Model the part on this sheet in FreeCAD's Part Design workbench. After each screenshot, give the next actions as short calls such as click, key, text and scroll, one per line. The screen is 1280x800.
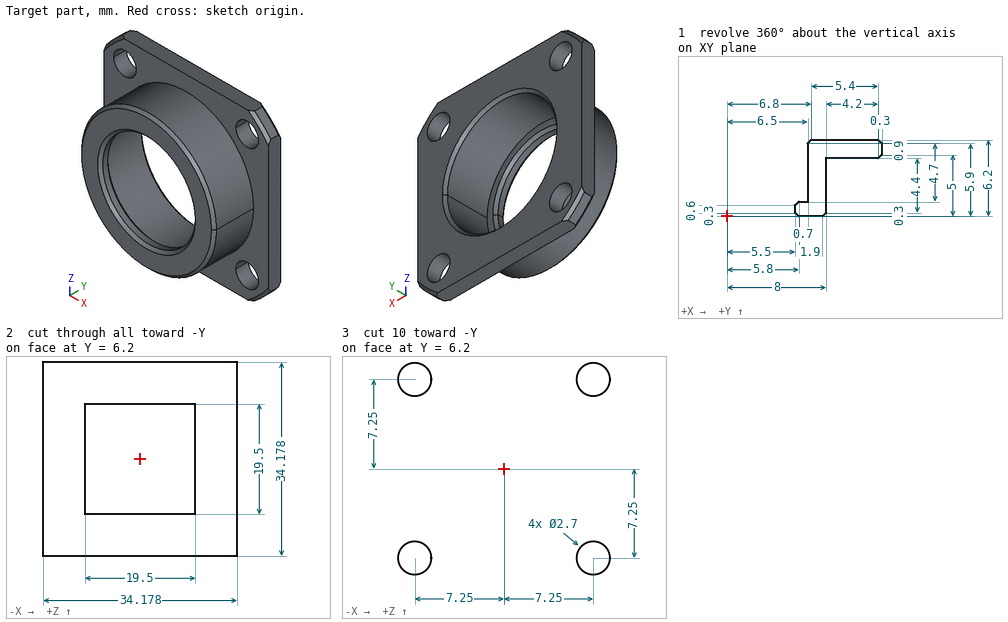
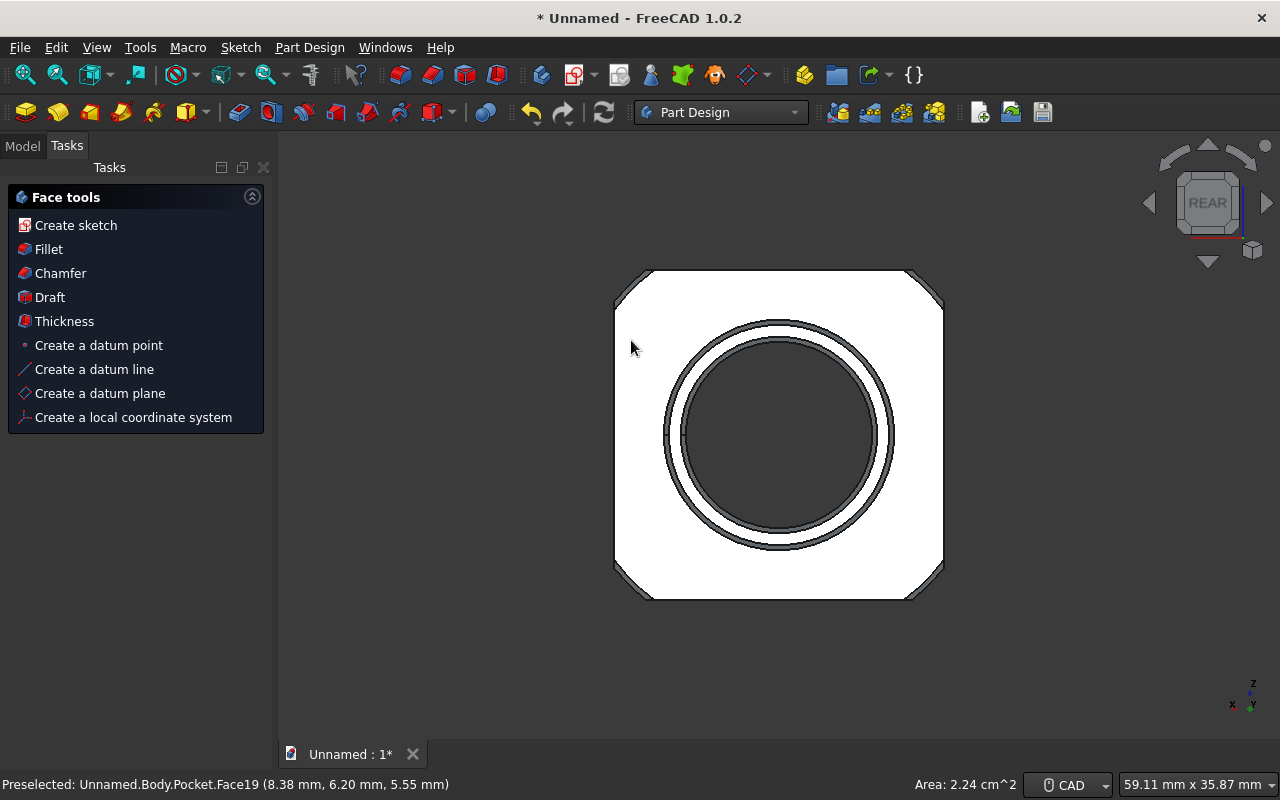
click(574, 76)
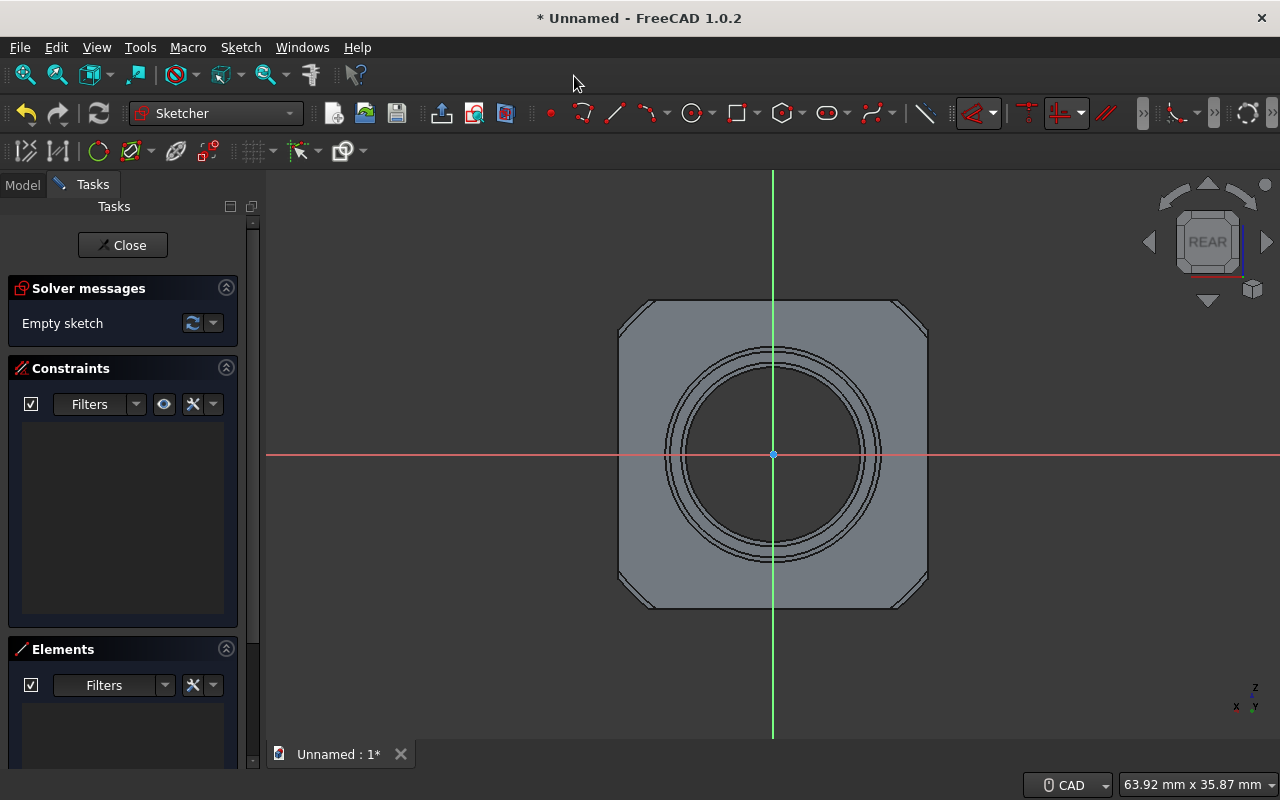
click(692, 114)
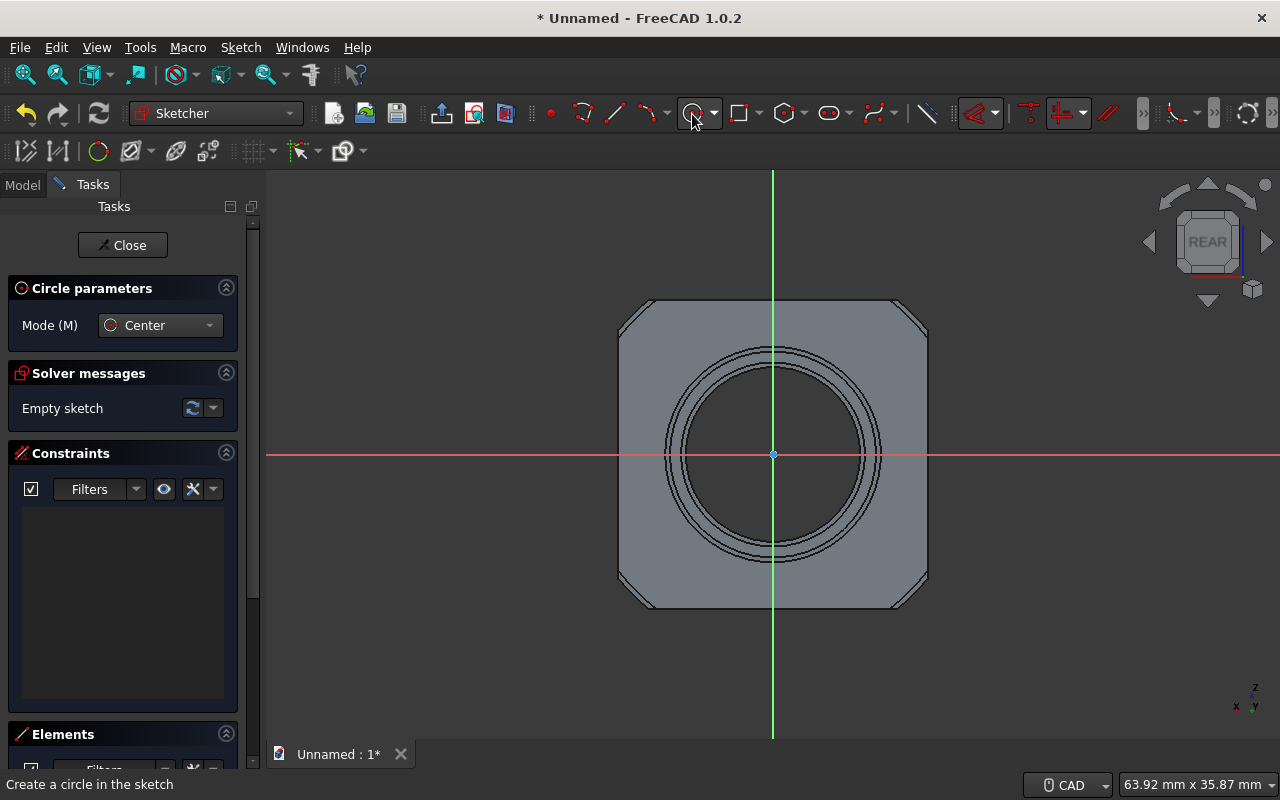
click(888, 570)
click(903, 554)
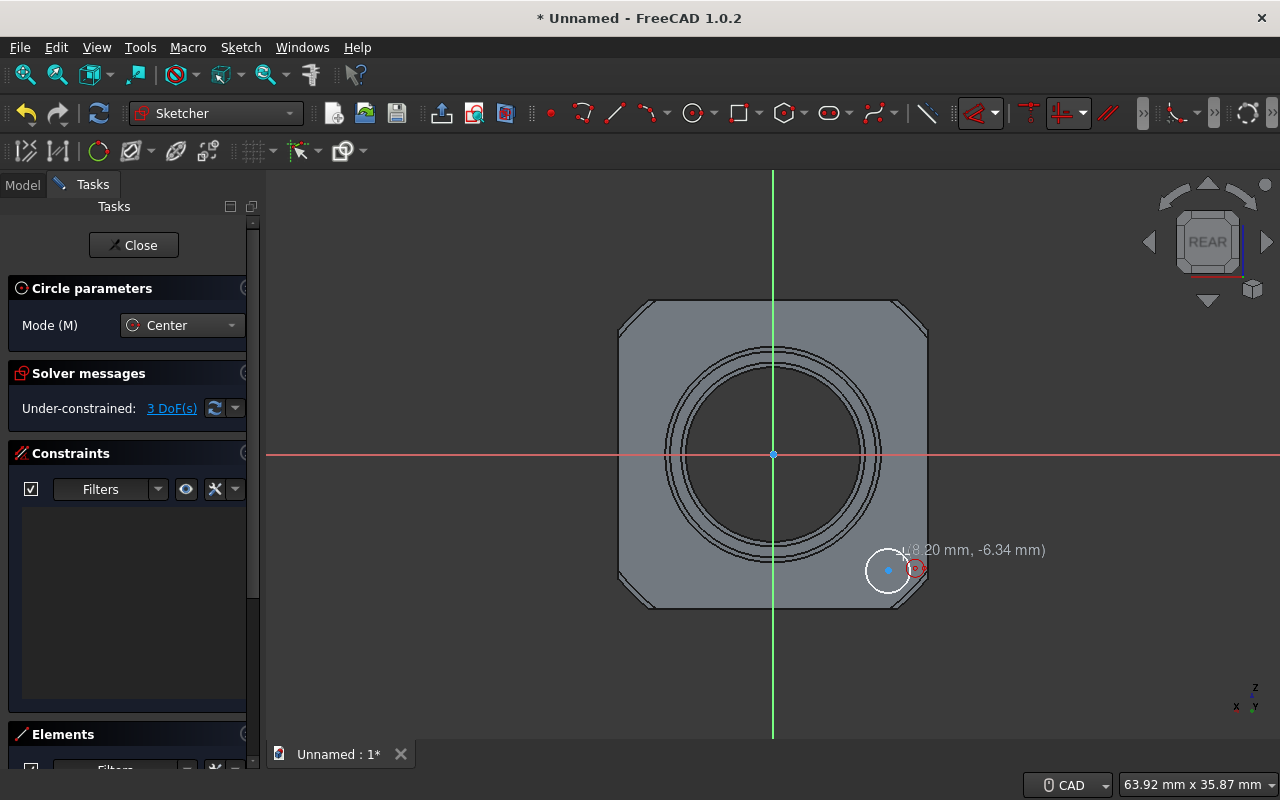
click(658, 570)
click(673, 554)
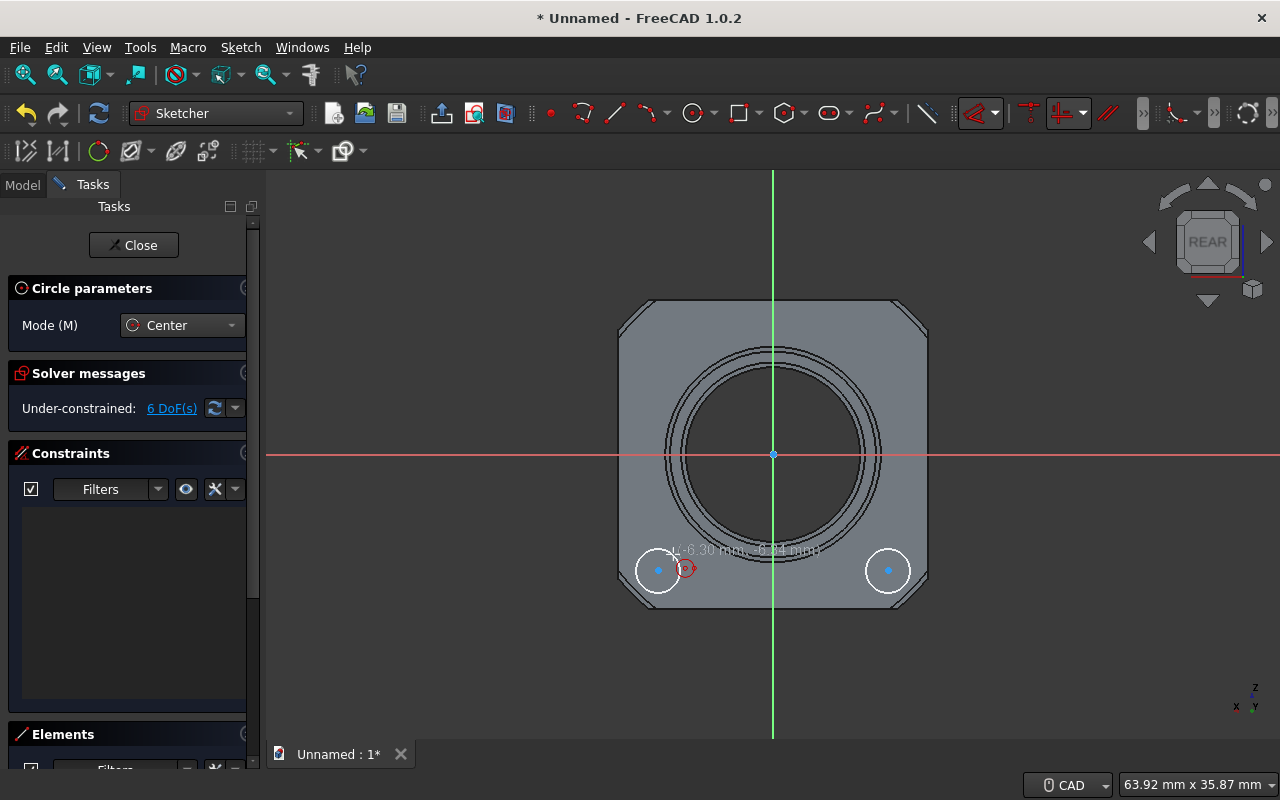
click(658, 339)
click(673, 324)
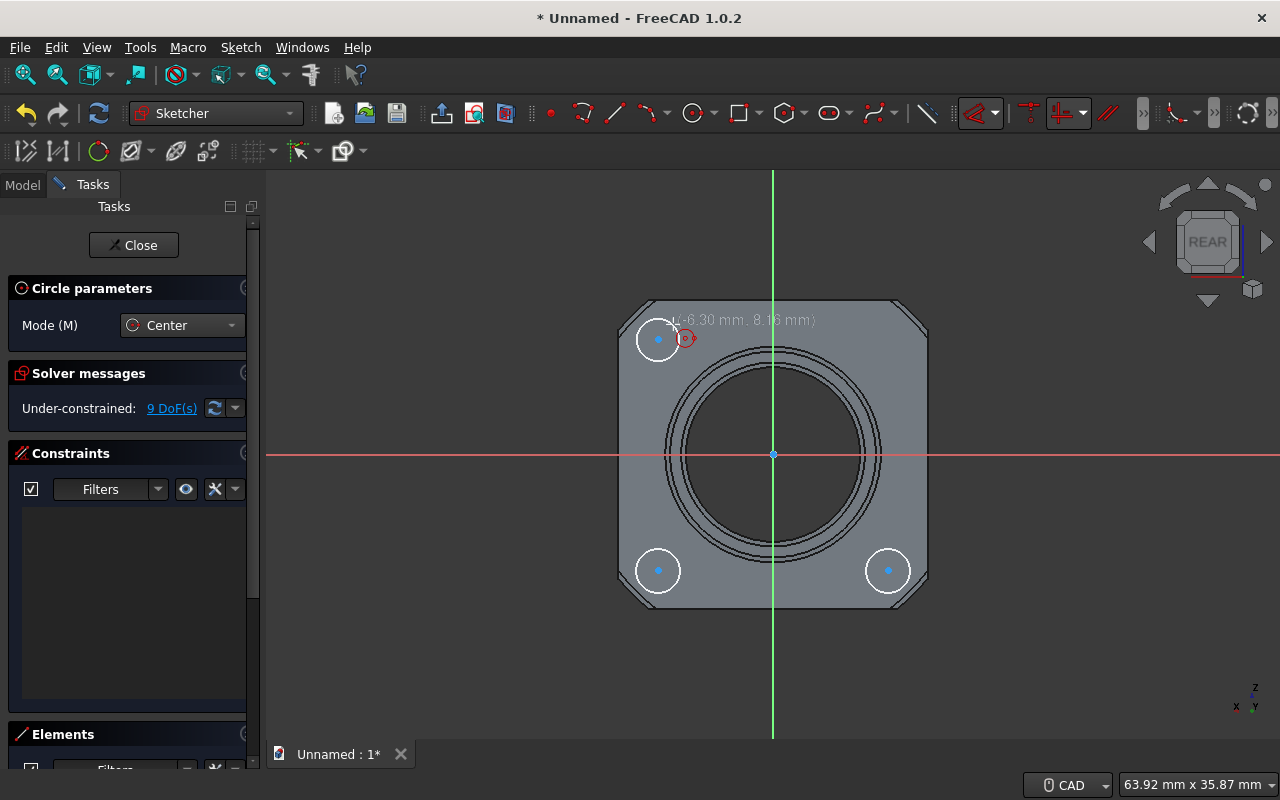
click(888, 339)
click(903, 324)
key(Escape)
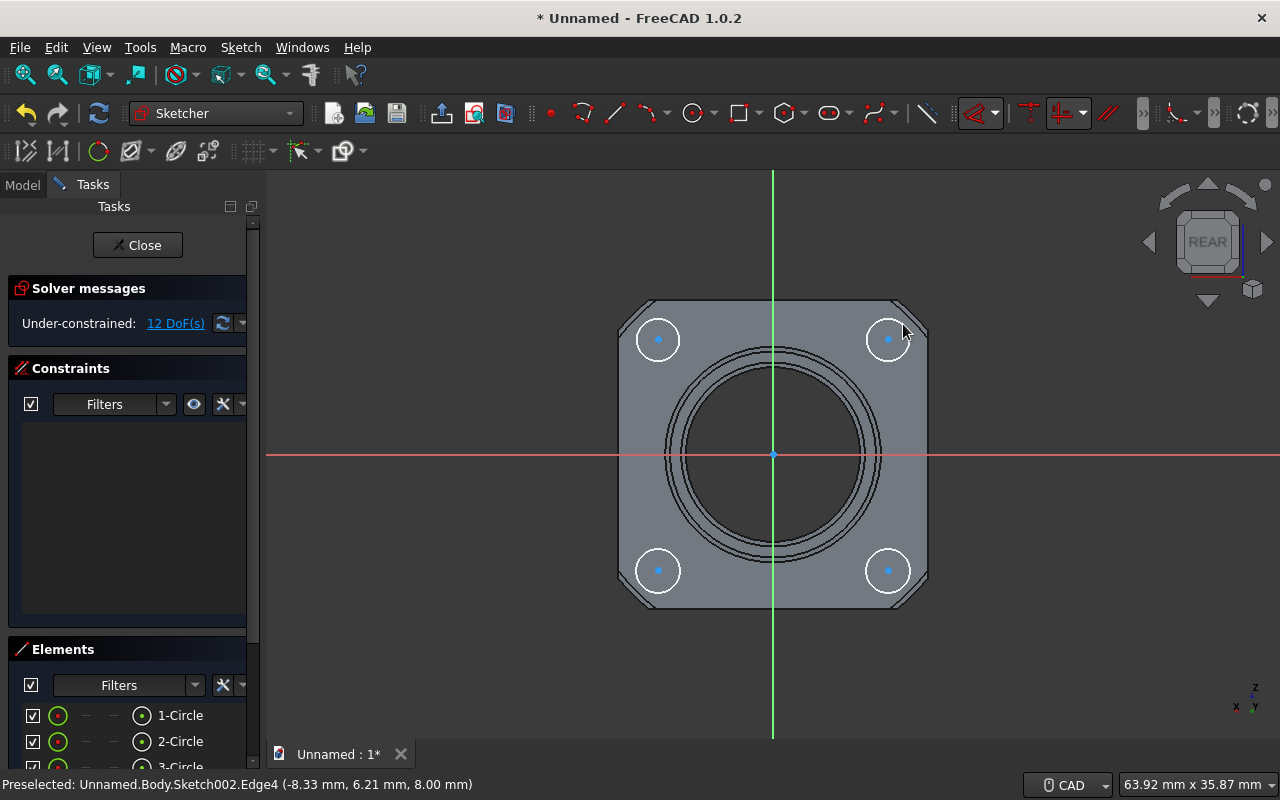
click(903, 555)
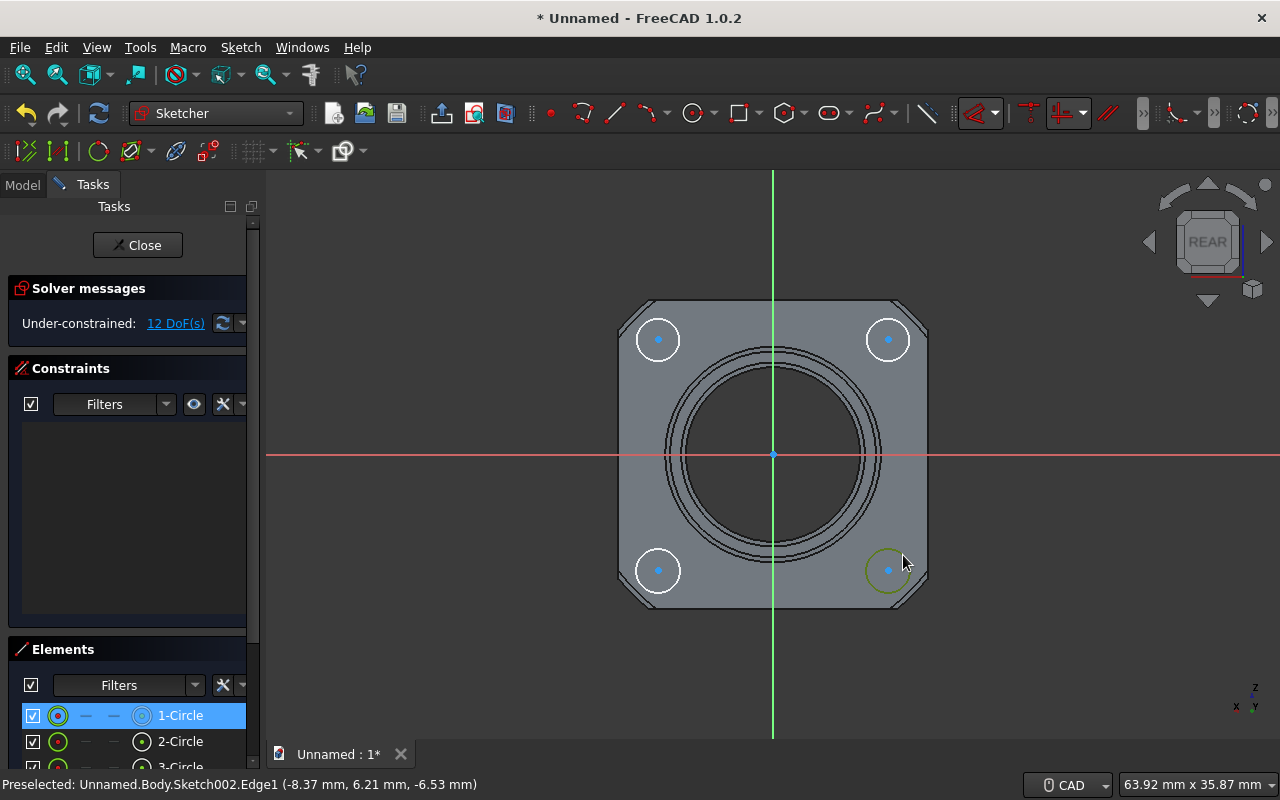
click(673, 555)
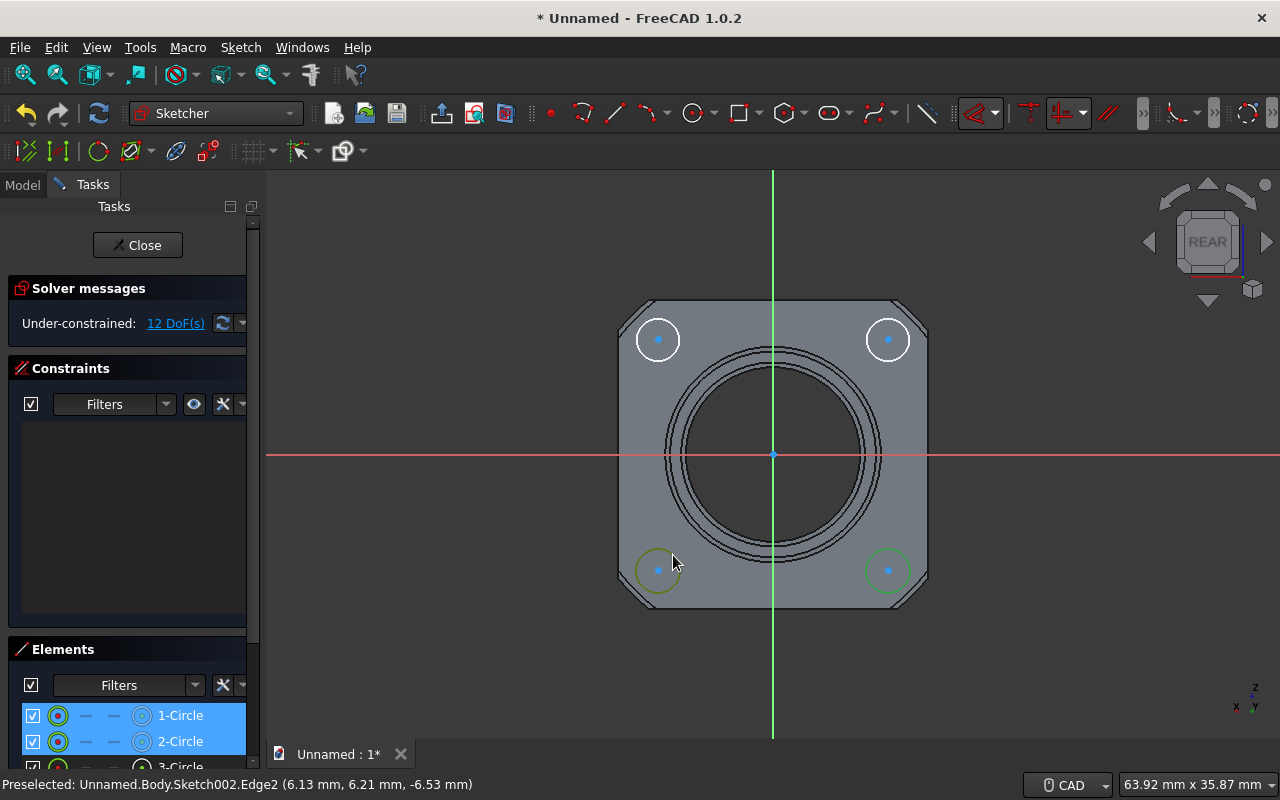
click(673, 325)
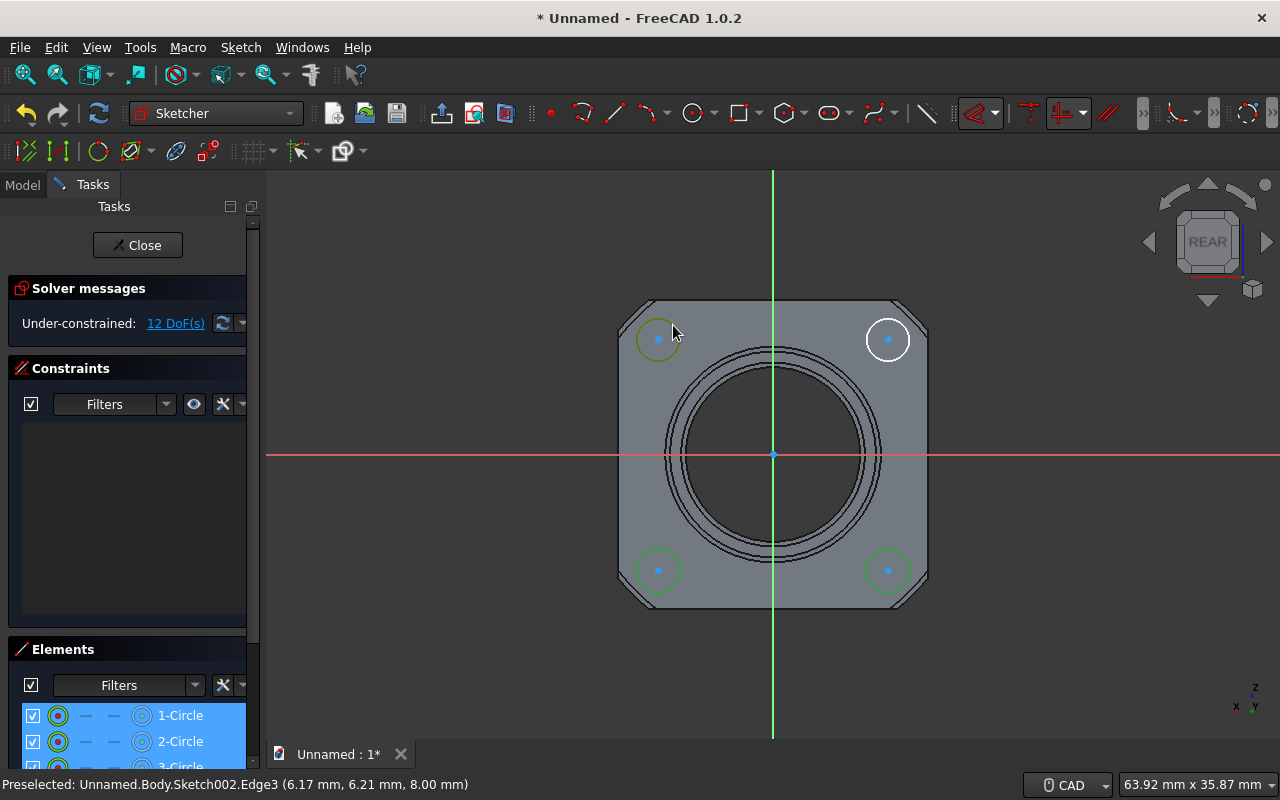
click(903, 325)